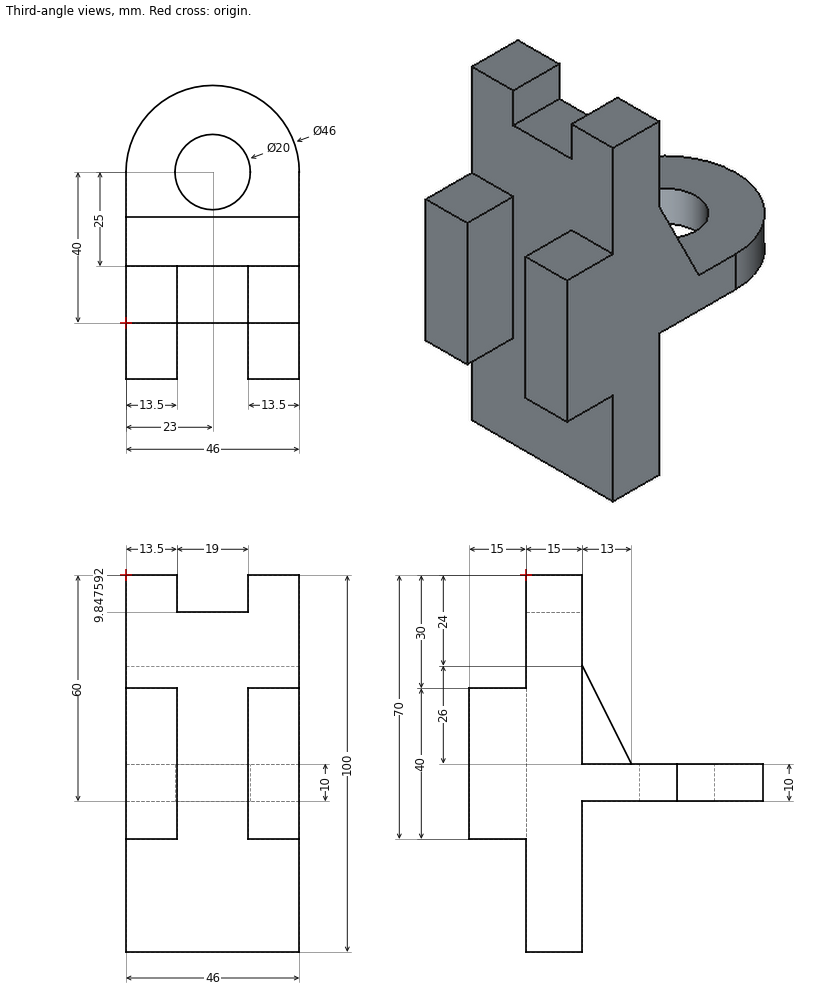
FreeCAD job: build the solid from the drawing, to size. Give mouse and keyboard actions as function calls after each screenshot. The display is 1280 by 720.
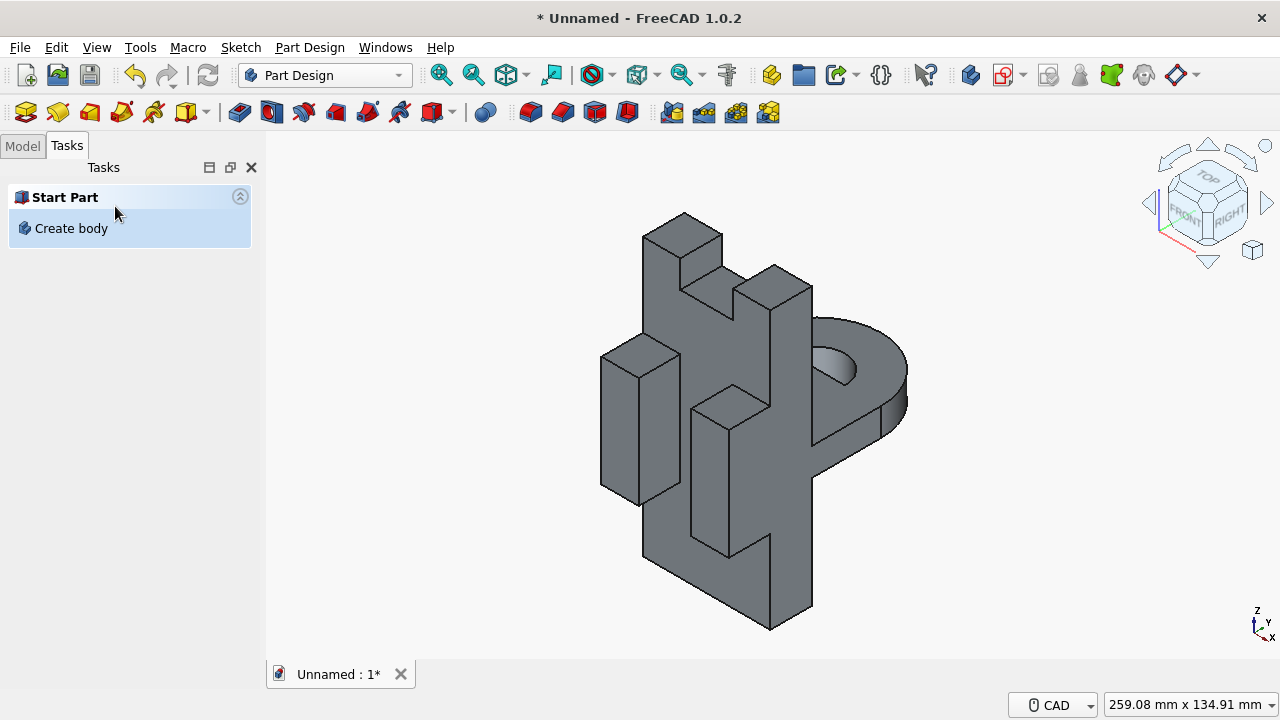
click(832, 402)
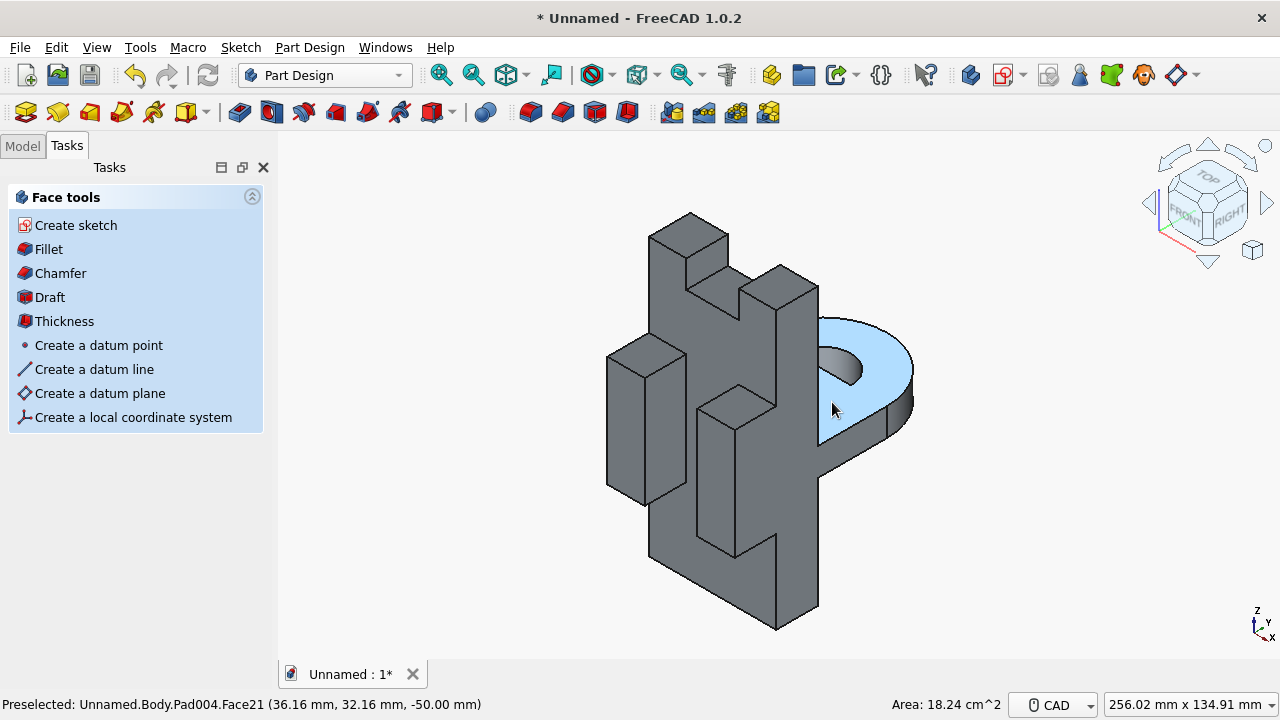
click(1004, 76)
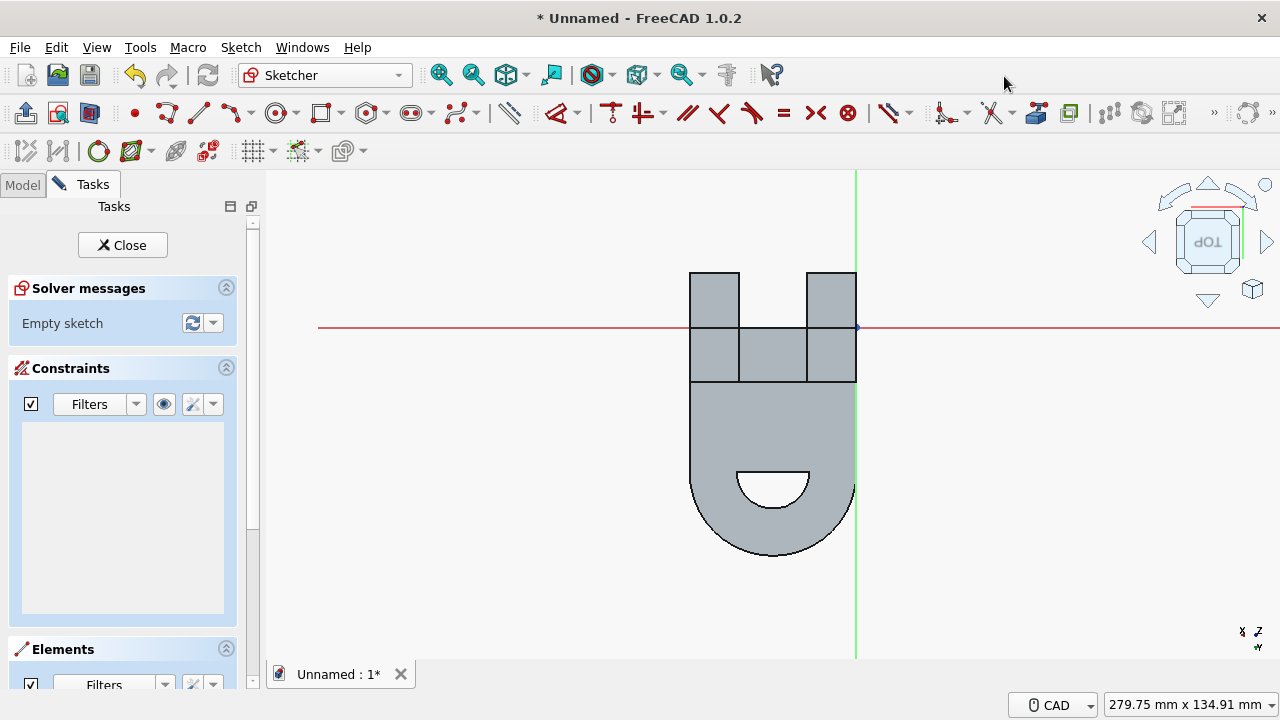
key(q)
key(s)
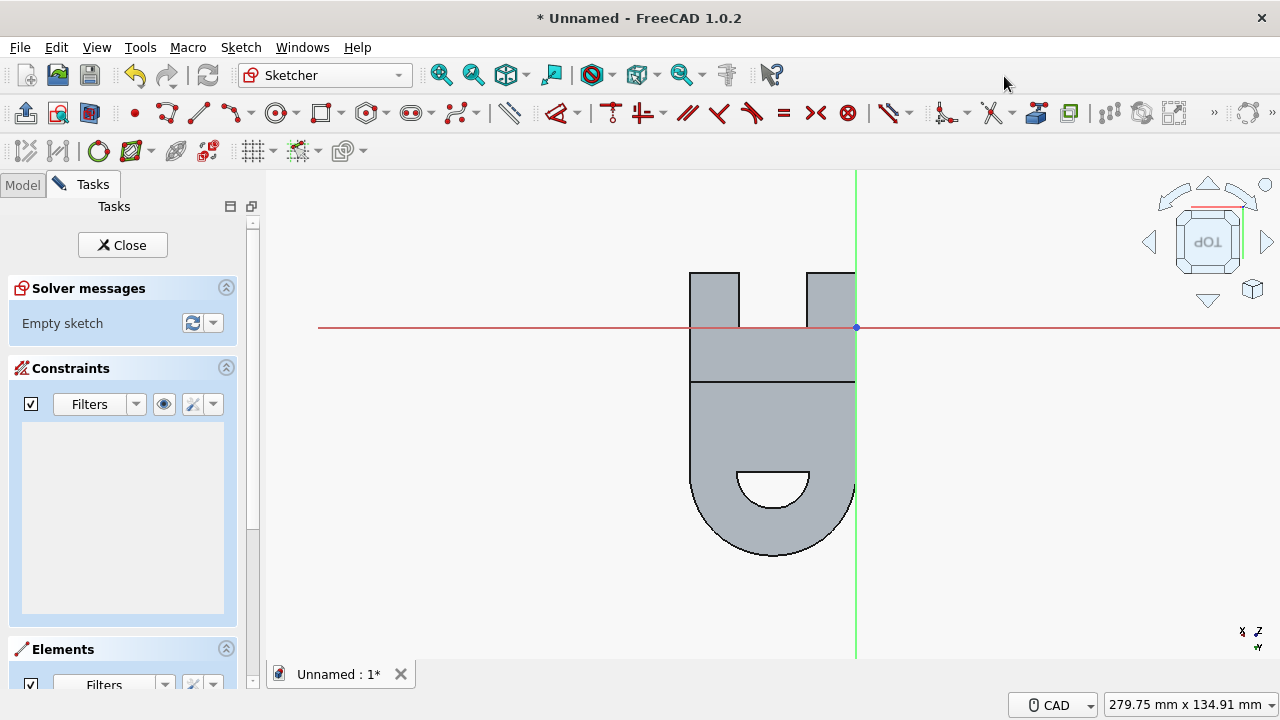
scroll(795, 491, up, 7)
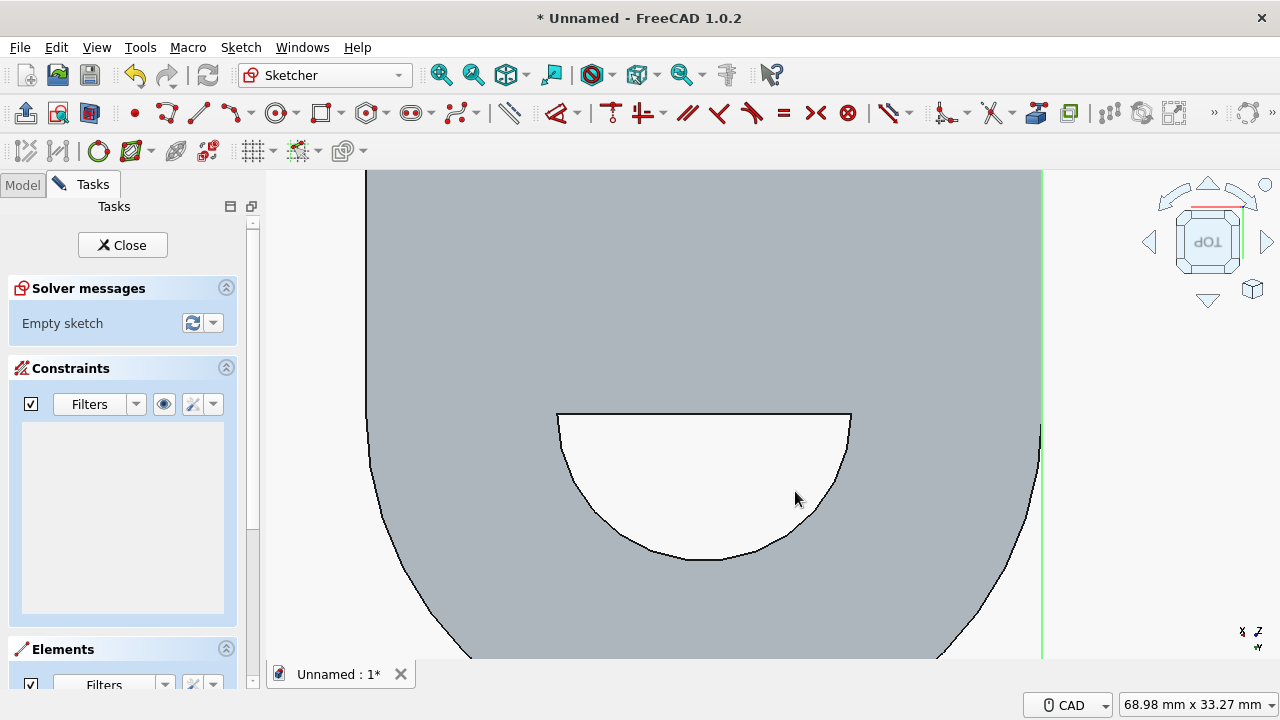
click(276, 114)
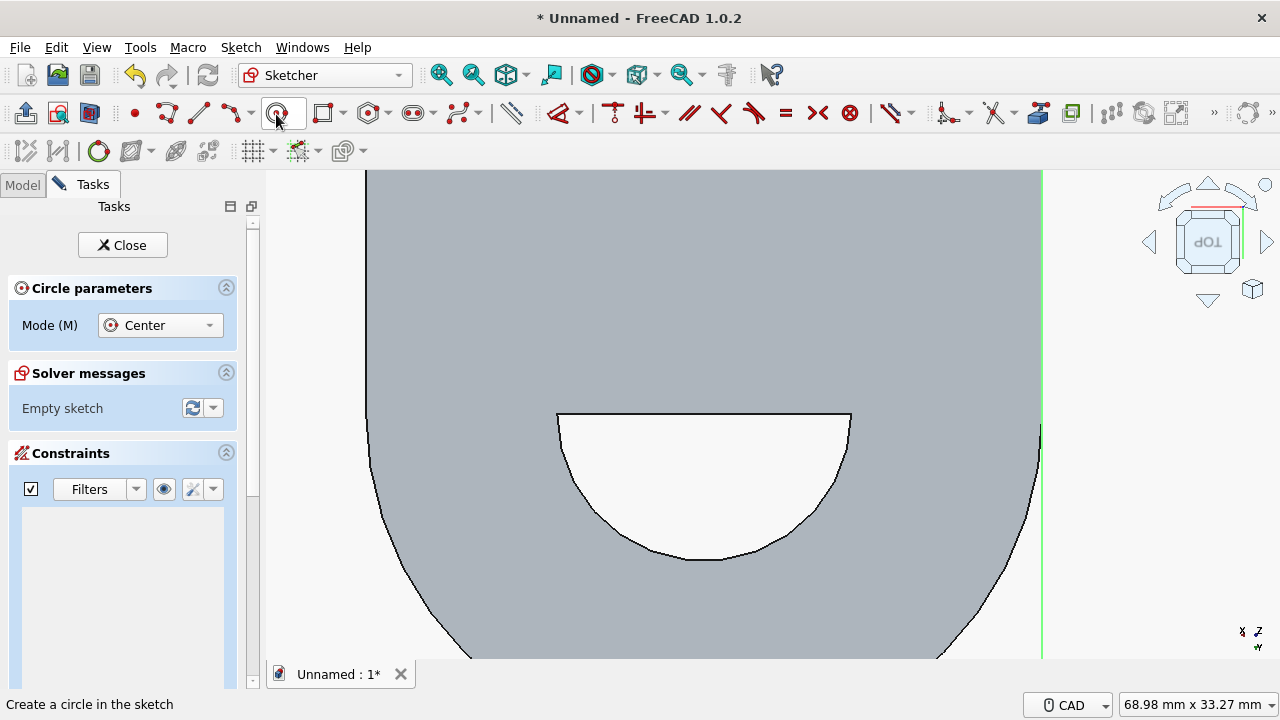
click(704, 414)
move(808, 310)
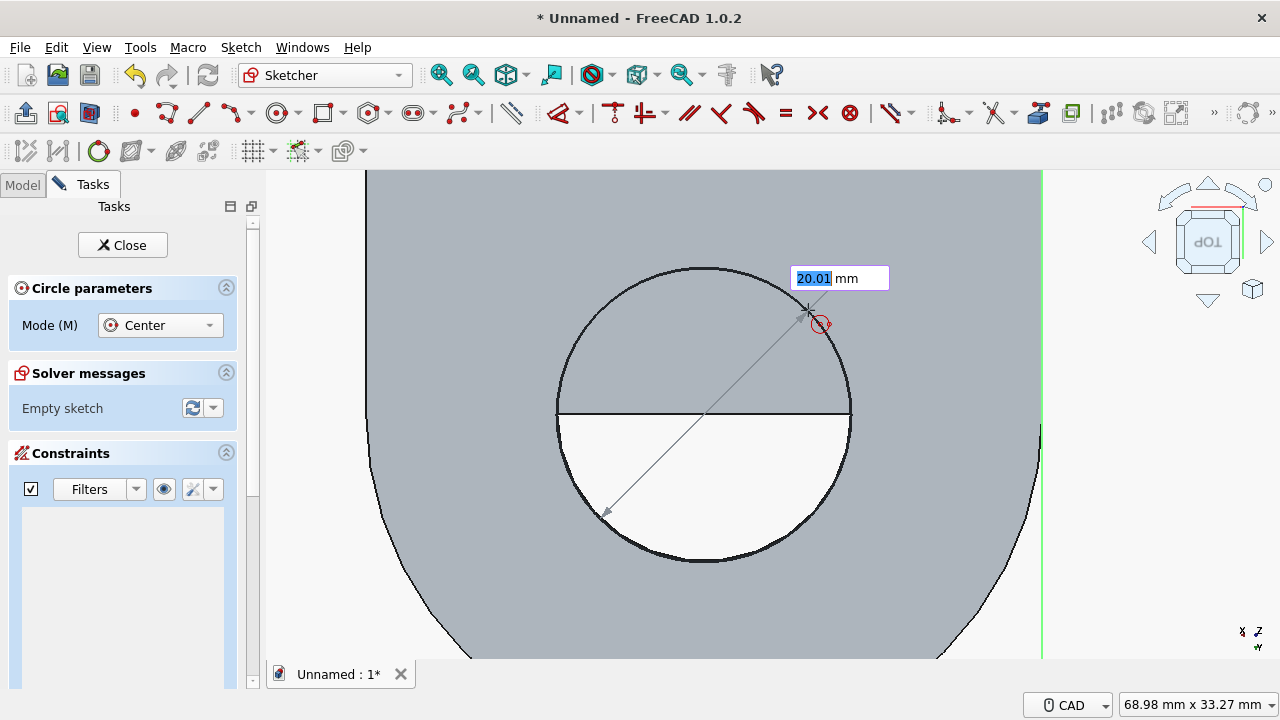
text(20)
key(Return)
key(Escape)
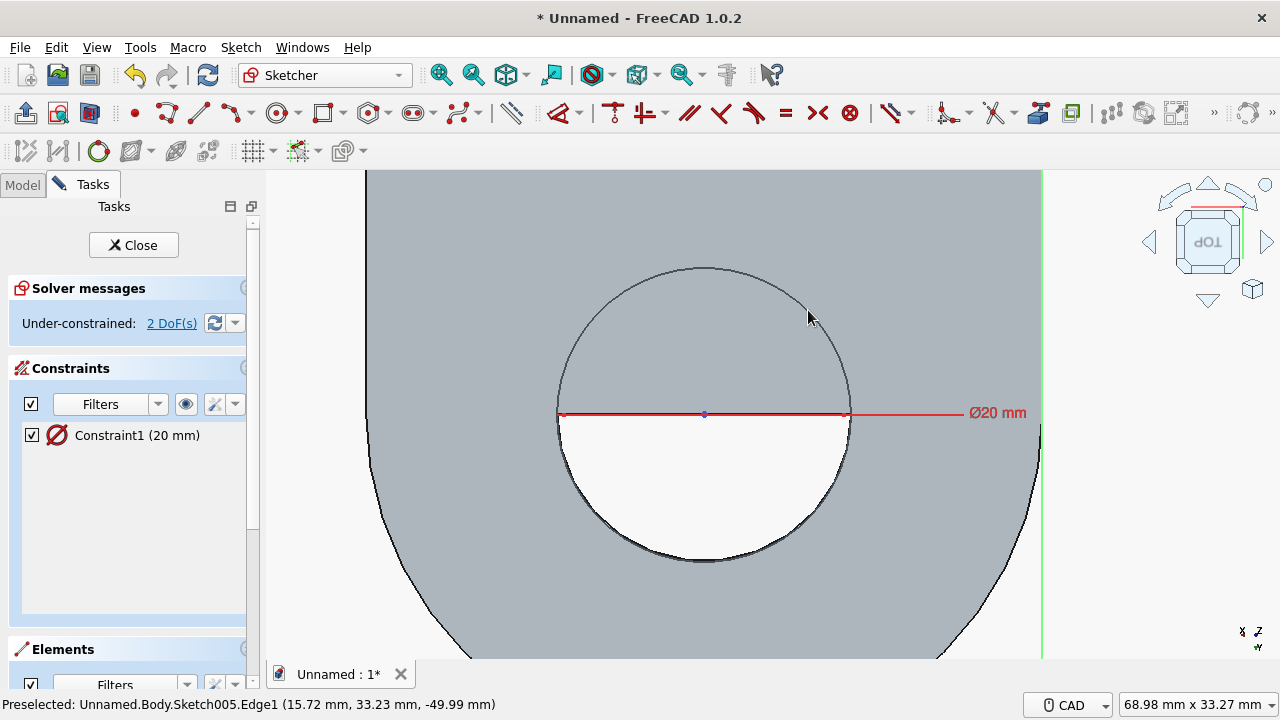
key(d)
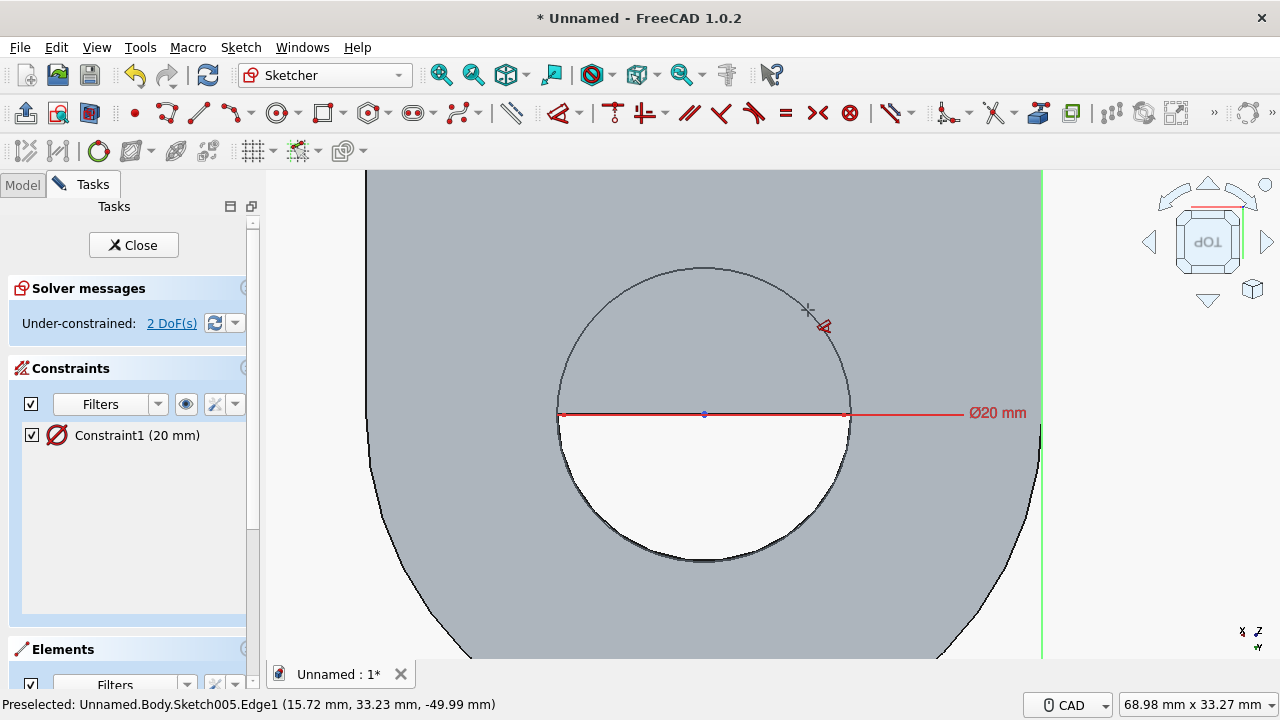
click(704, 415)
click(873, 449)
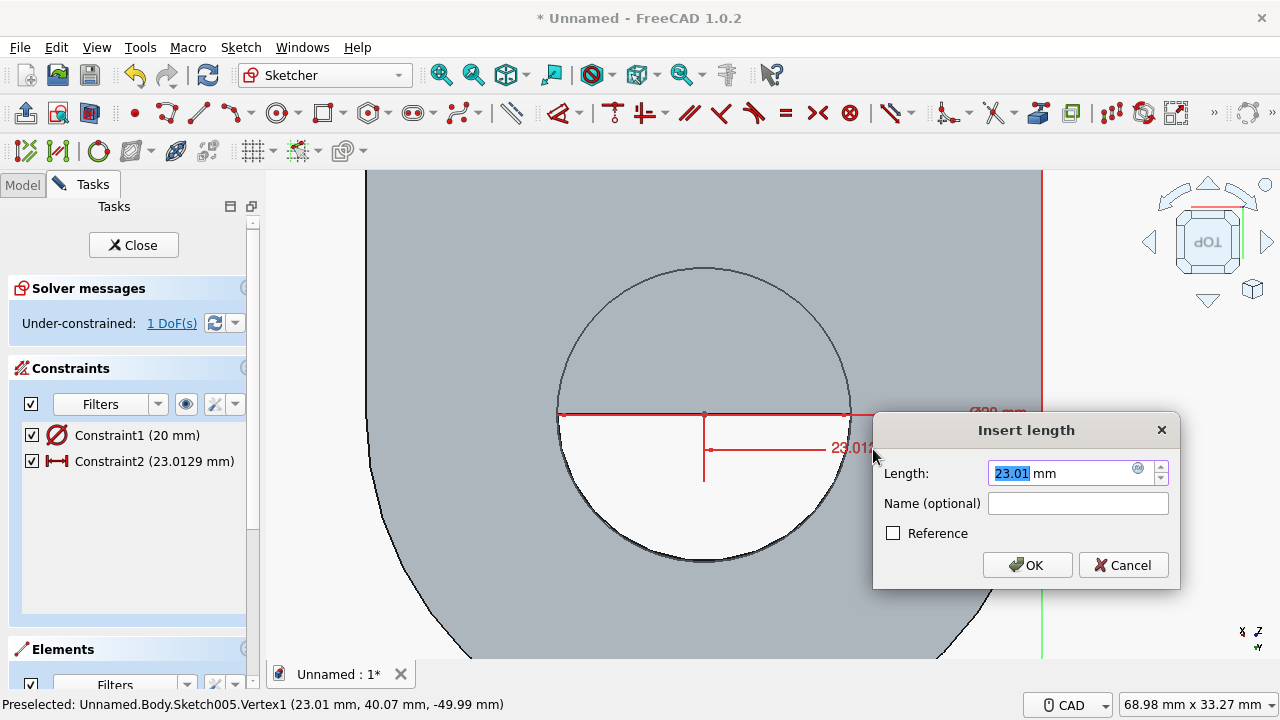
text(23)
key(Return)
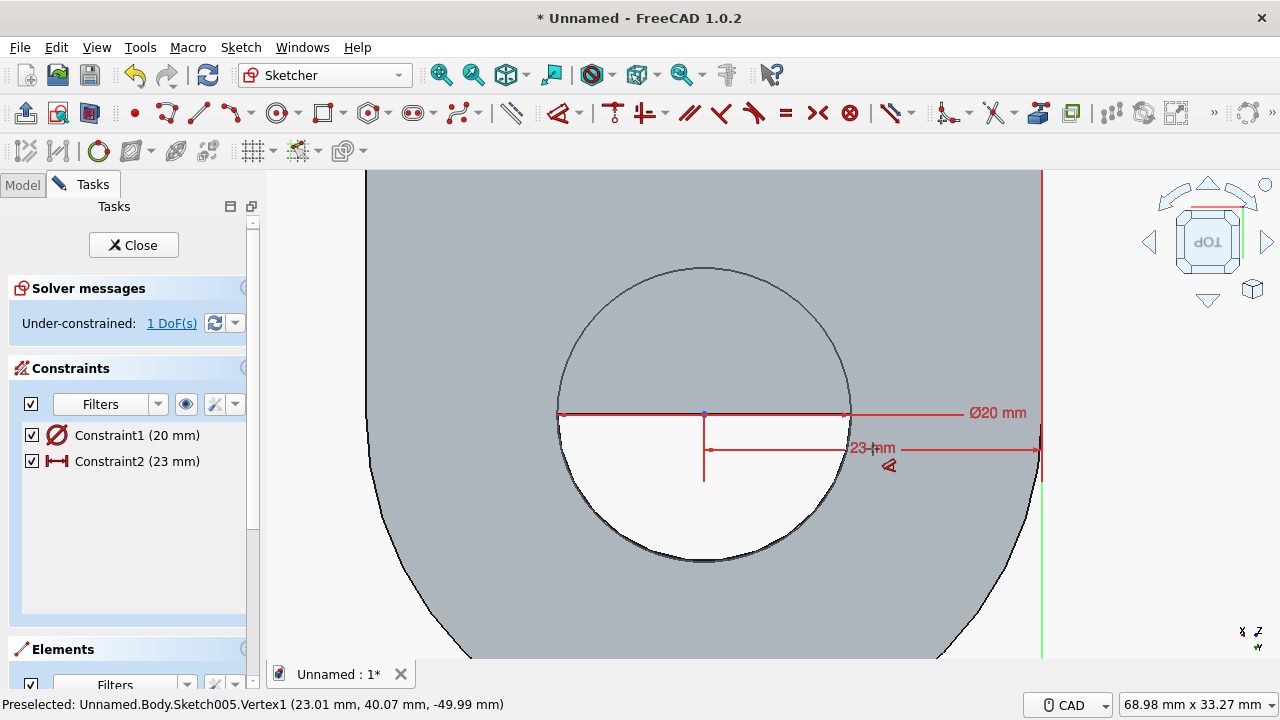
click(704, 415)
click(1076, 306)